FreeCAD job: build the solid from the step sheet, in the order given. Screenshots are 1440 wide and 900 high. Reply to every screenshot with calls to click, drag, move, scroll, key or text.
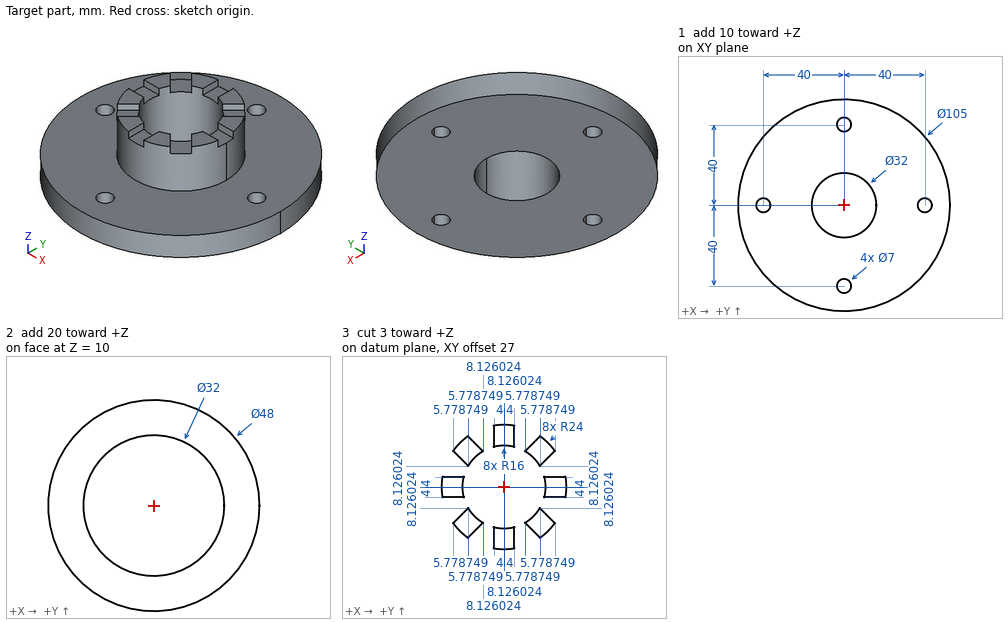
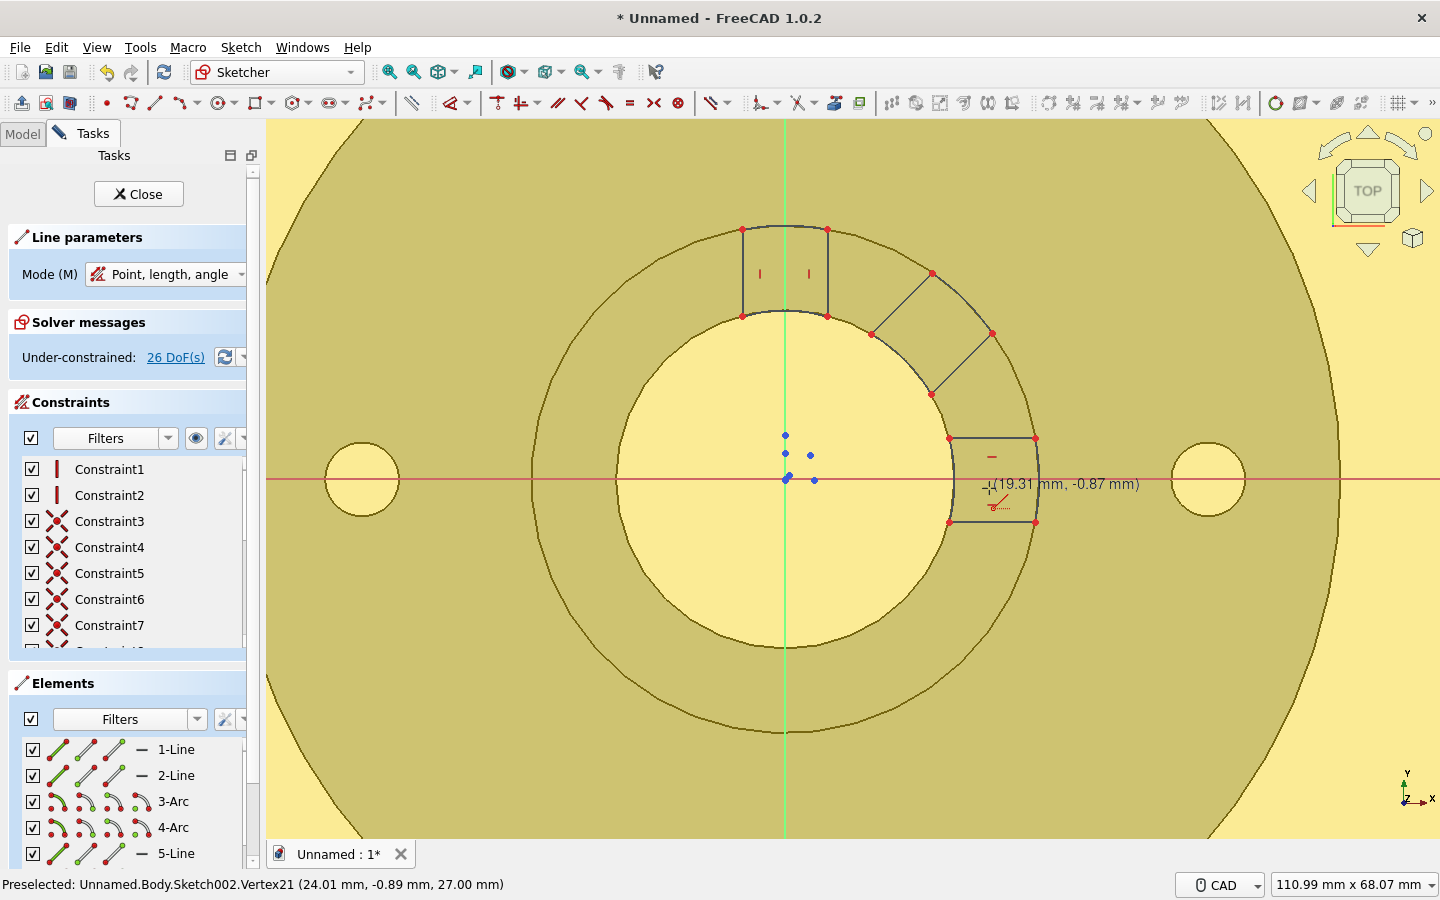
click(992, 626)
click(931, 565)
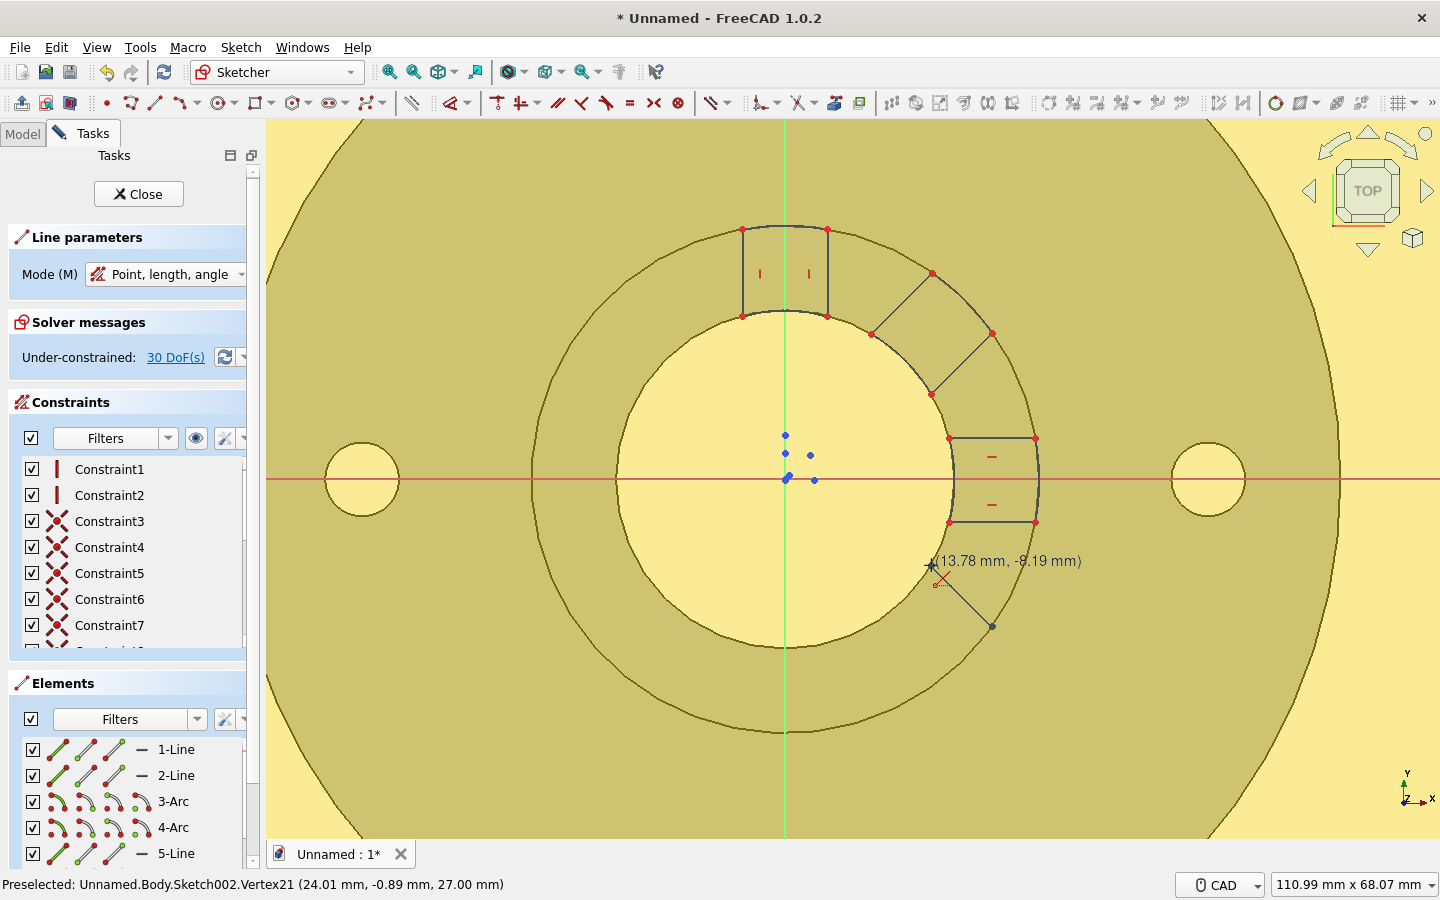
click(871, 625)
click(932, 686)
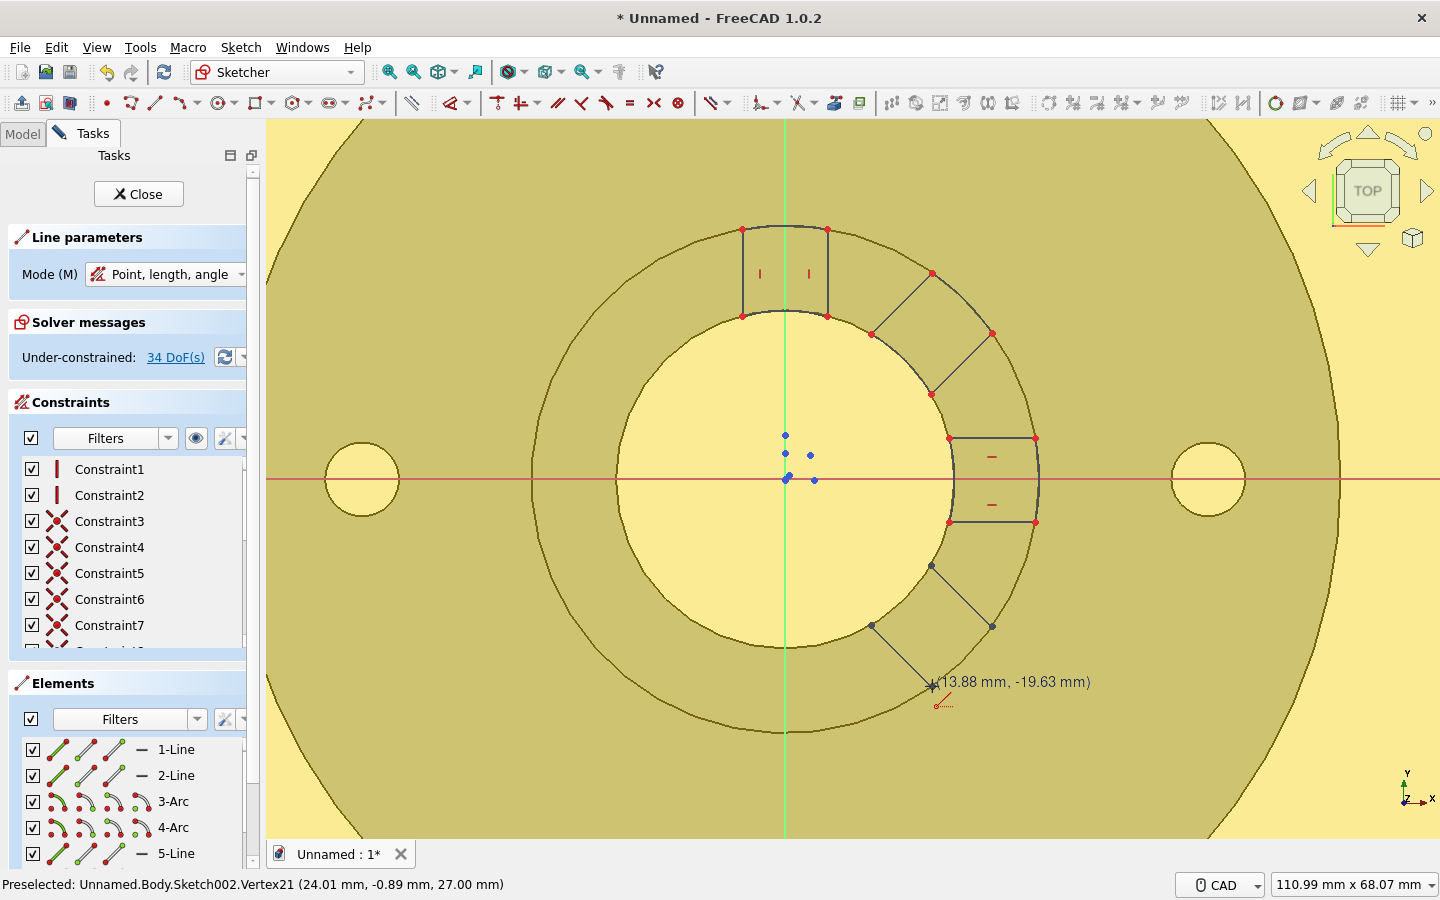
click(180, 104)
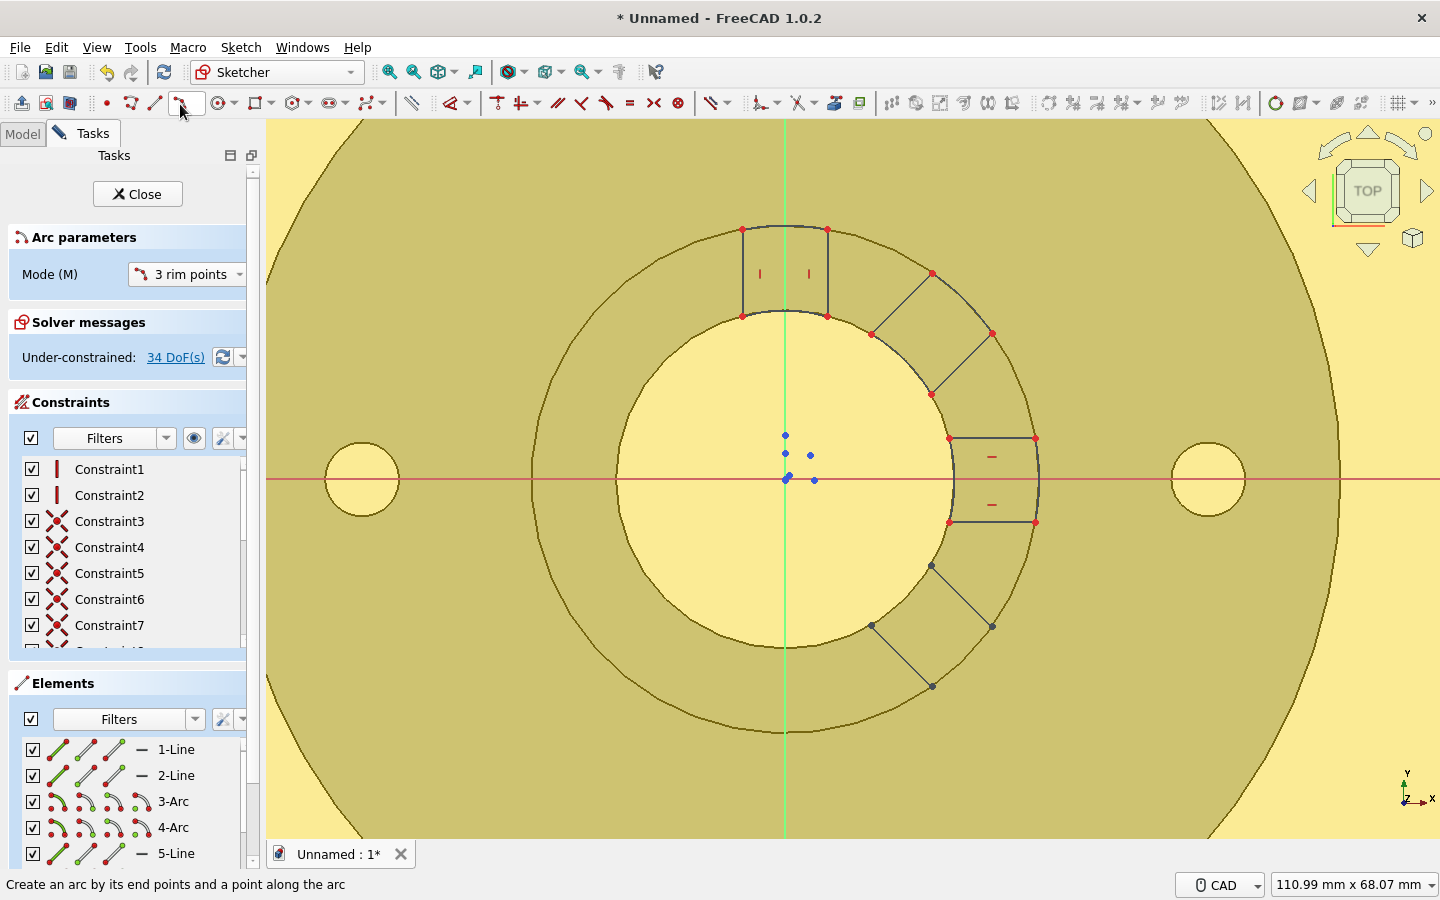
click(931, 566)
click(871, 626)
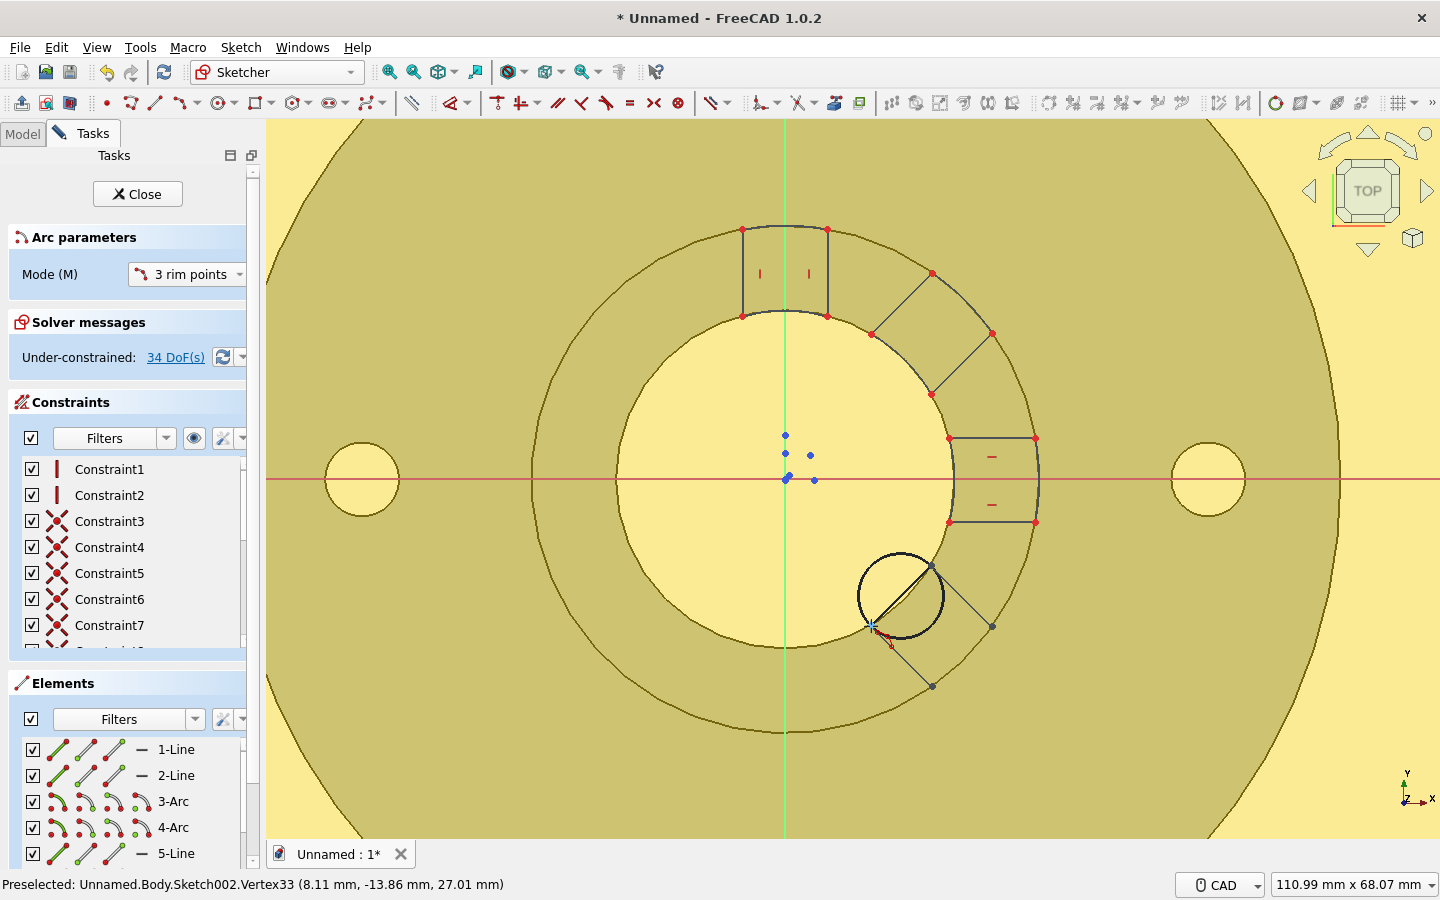
scroll(905, 599, up, 6)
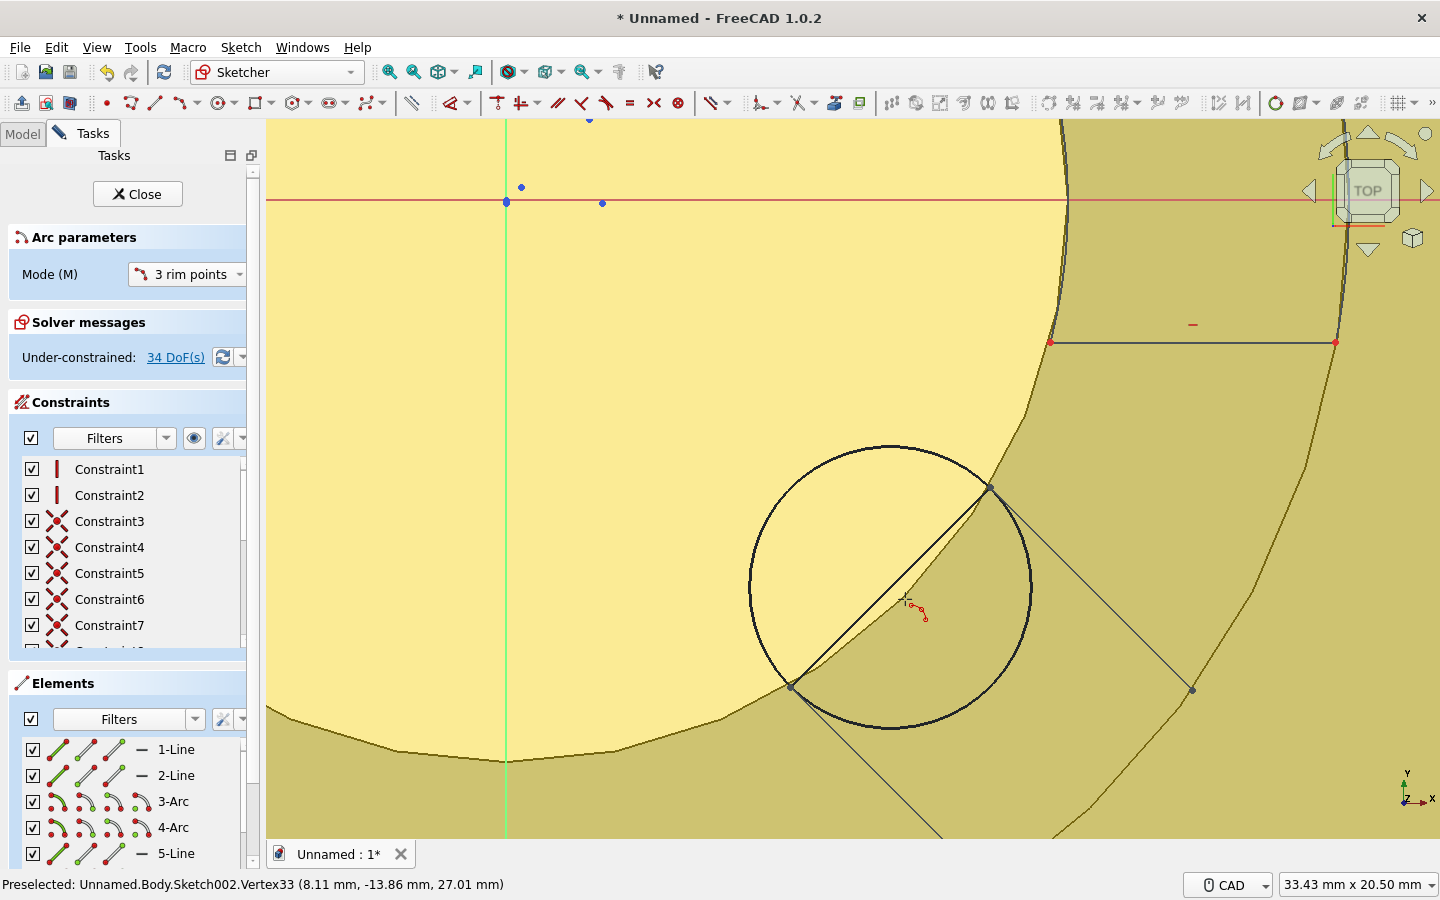
click(903, 598)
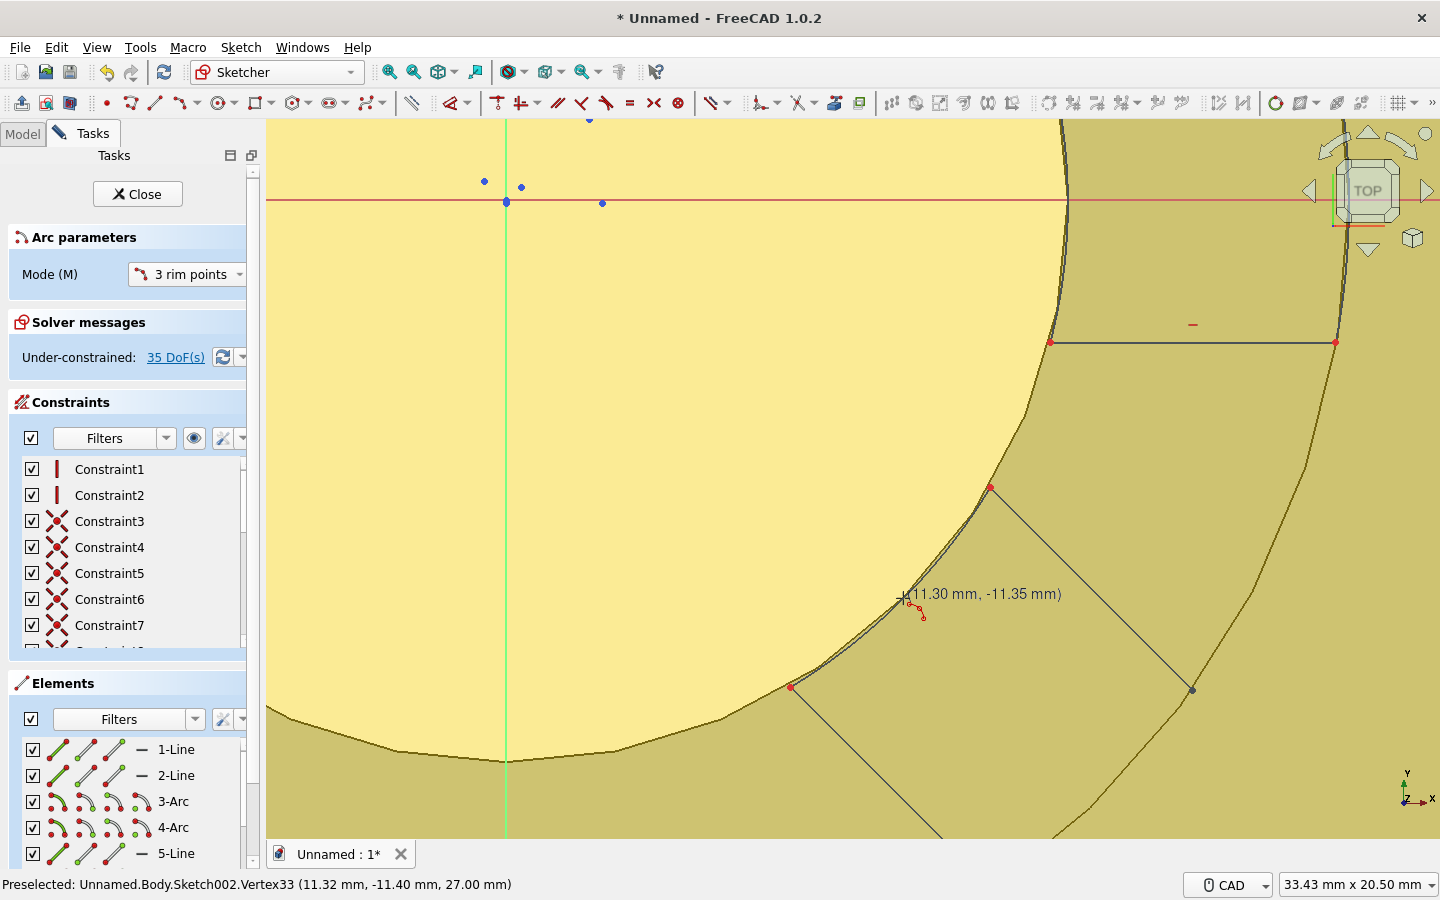
scroll(905, 599, down, 6)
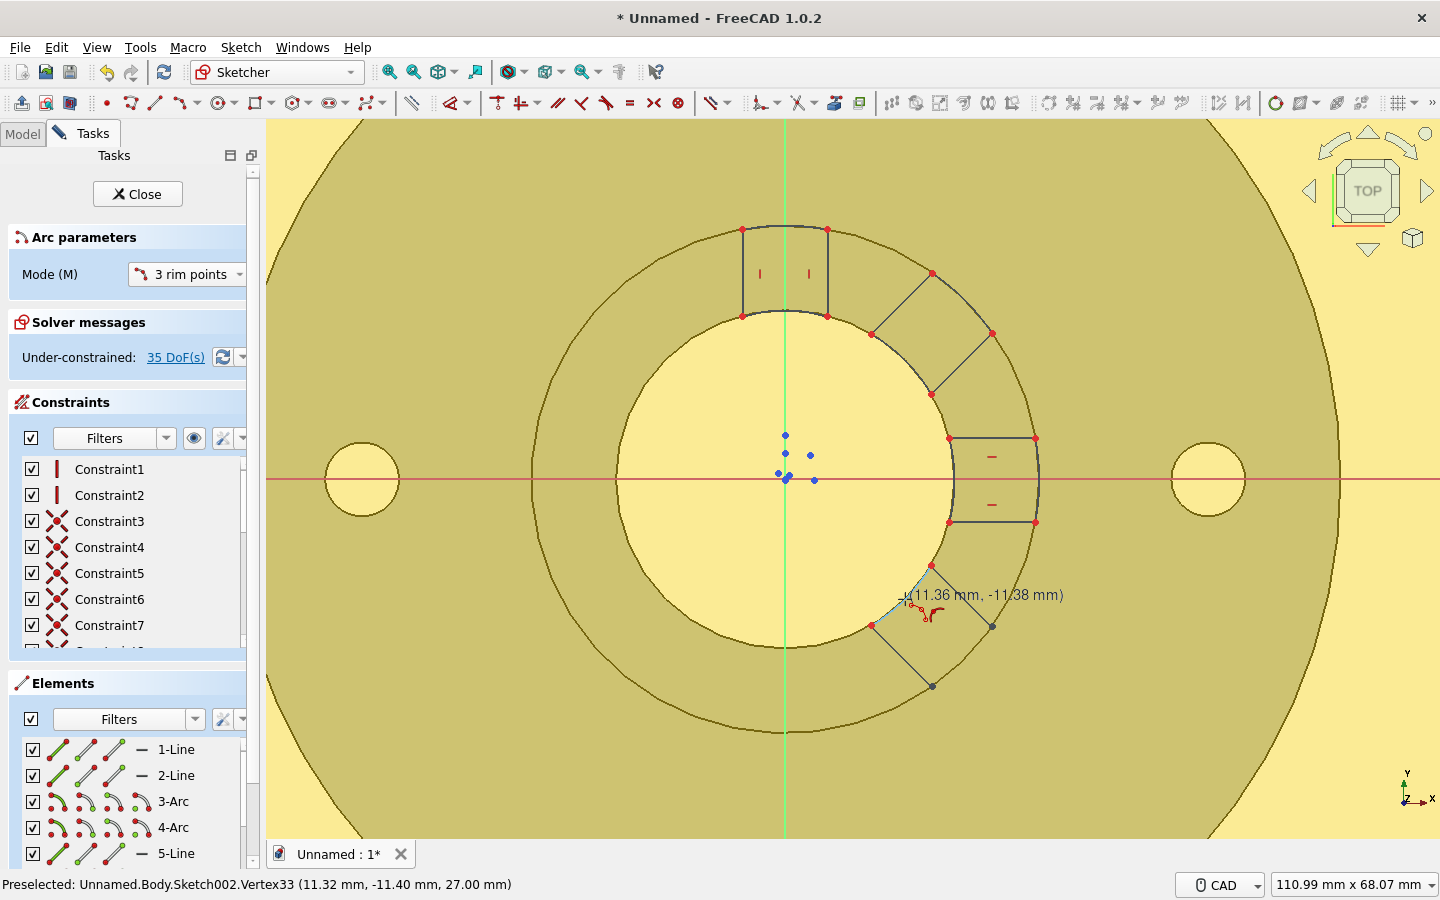
click(932, 687)
click(992, 627)